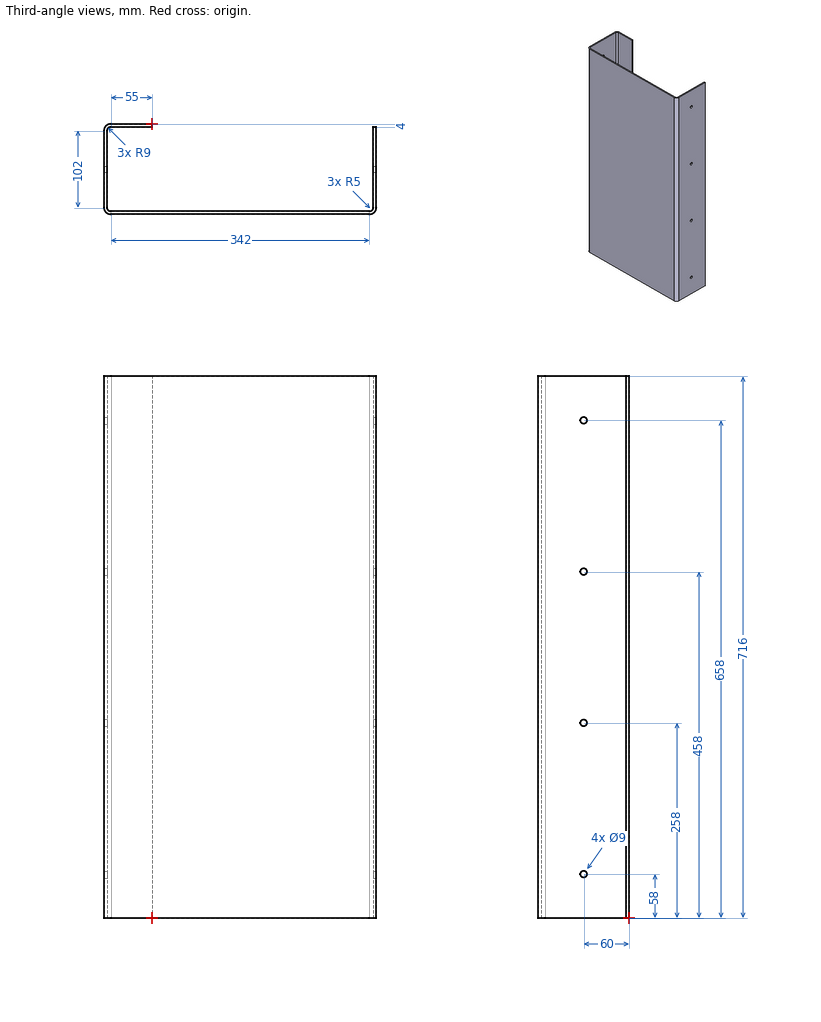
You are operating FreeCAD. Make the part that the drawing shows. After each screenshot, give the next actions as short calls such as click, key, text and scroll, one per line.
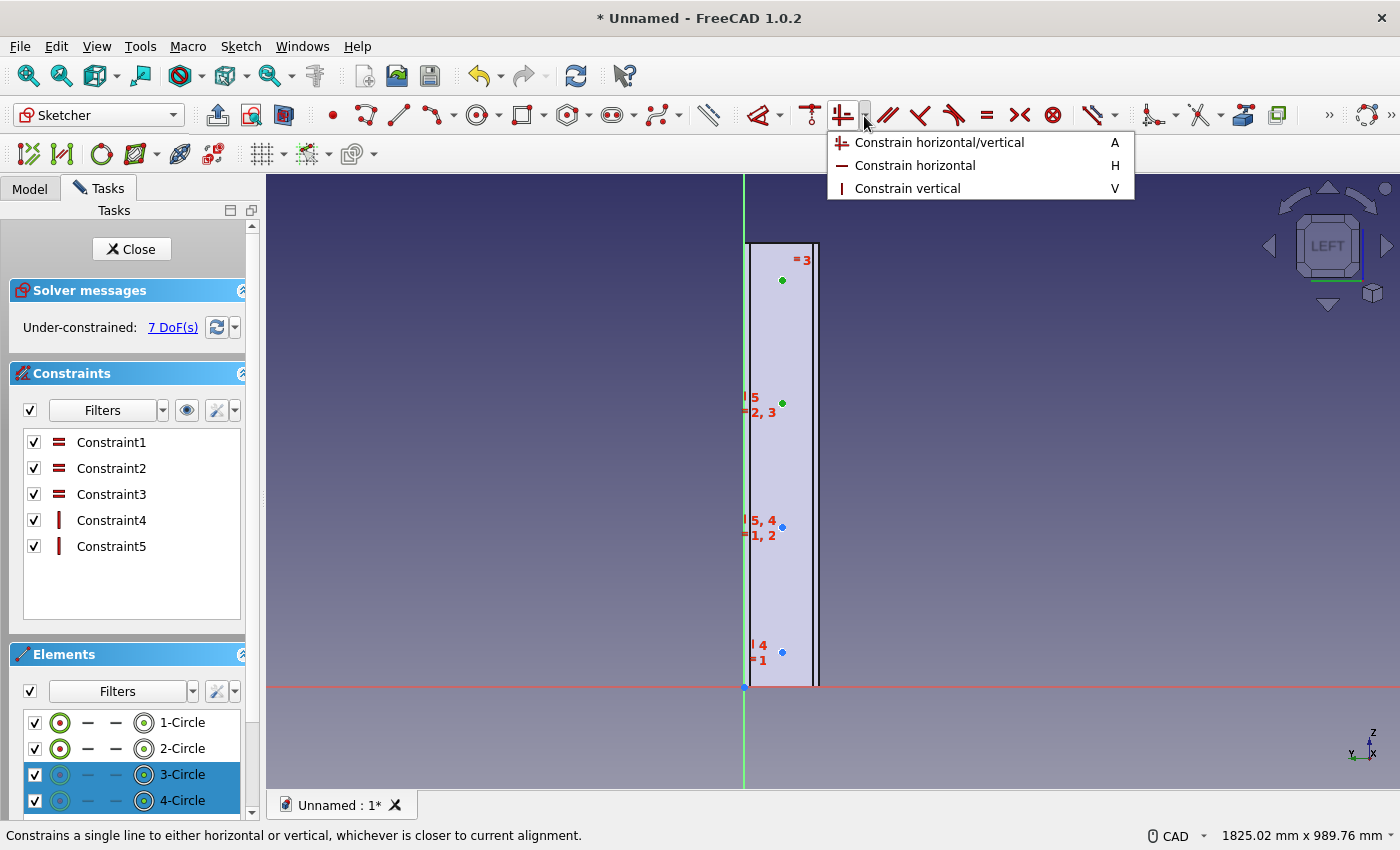
click(981, 188)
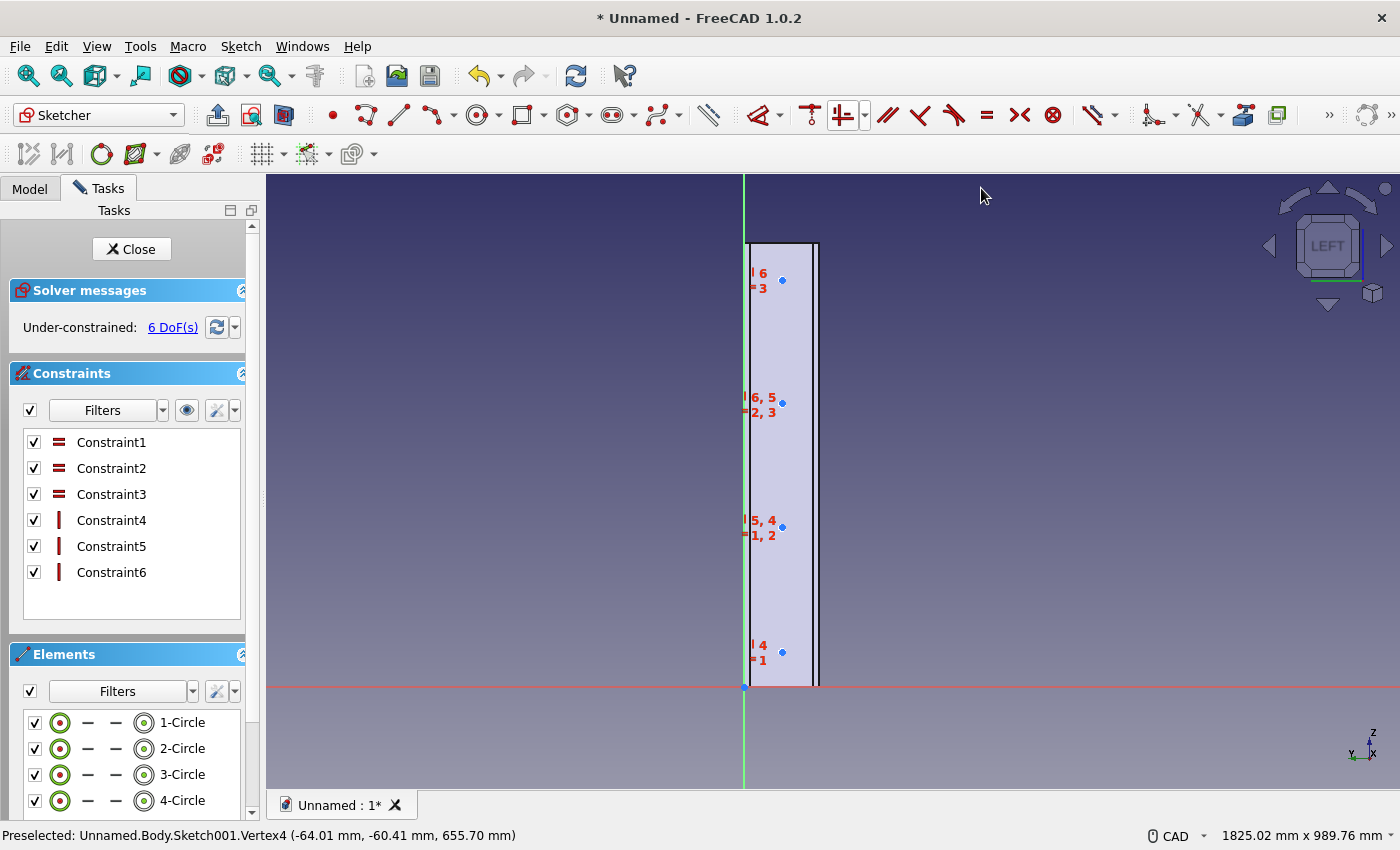
click(758, 116)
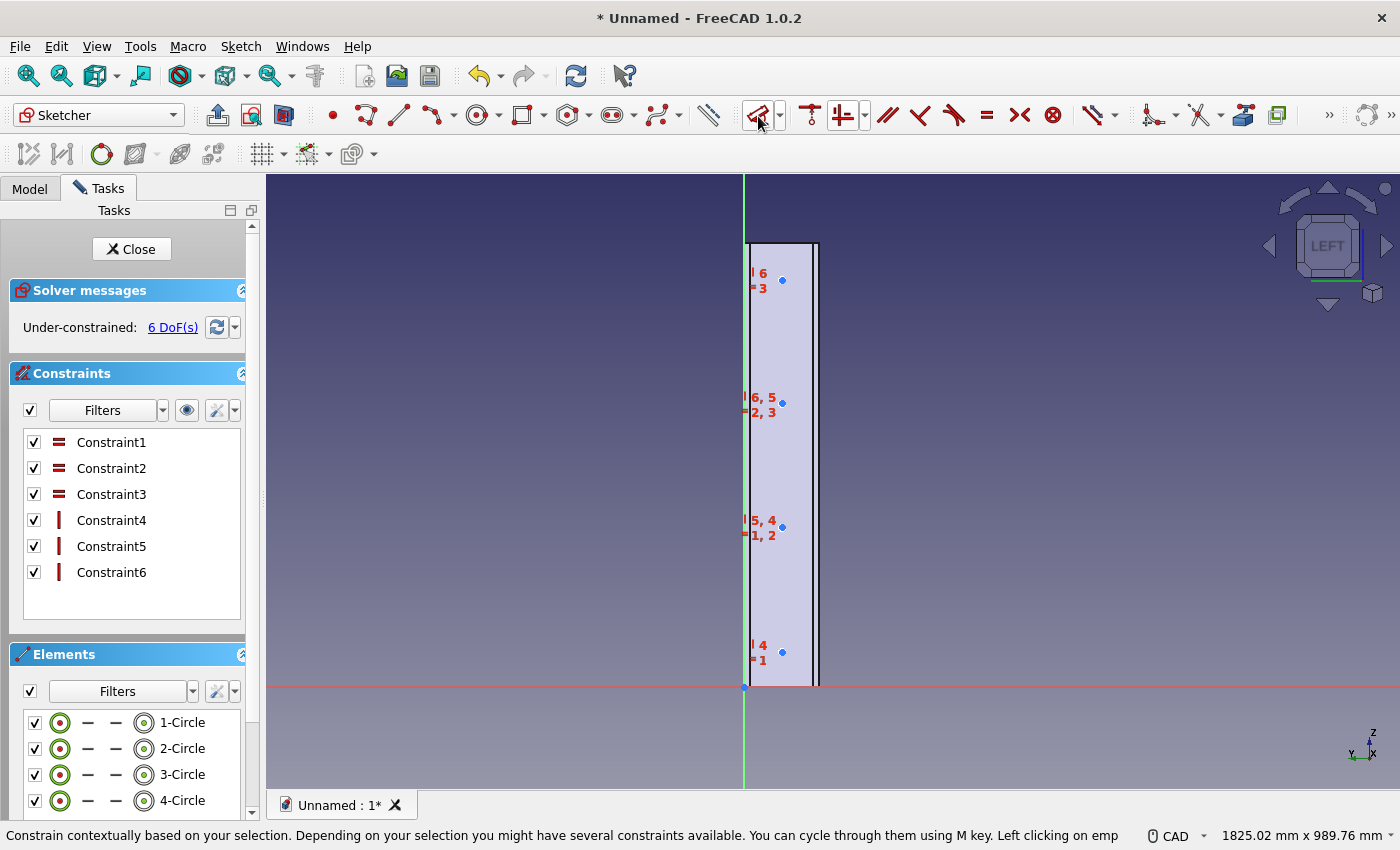
scroll(780, 650, up, 10)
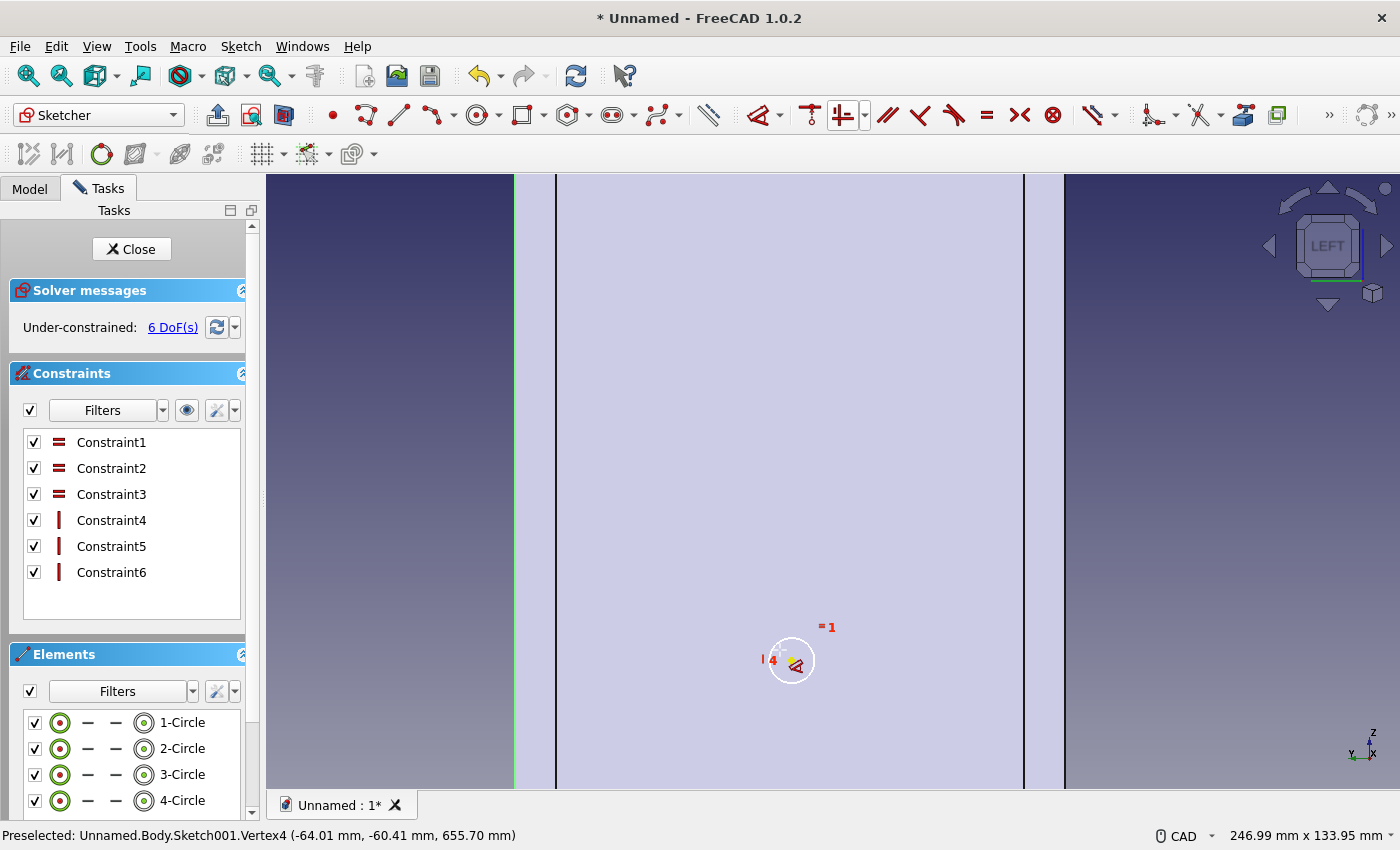
click(776, 645)
click(753, 623)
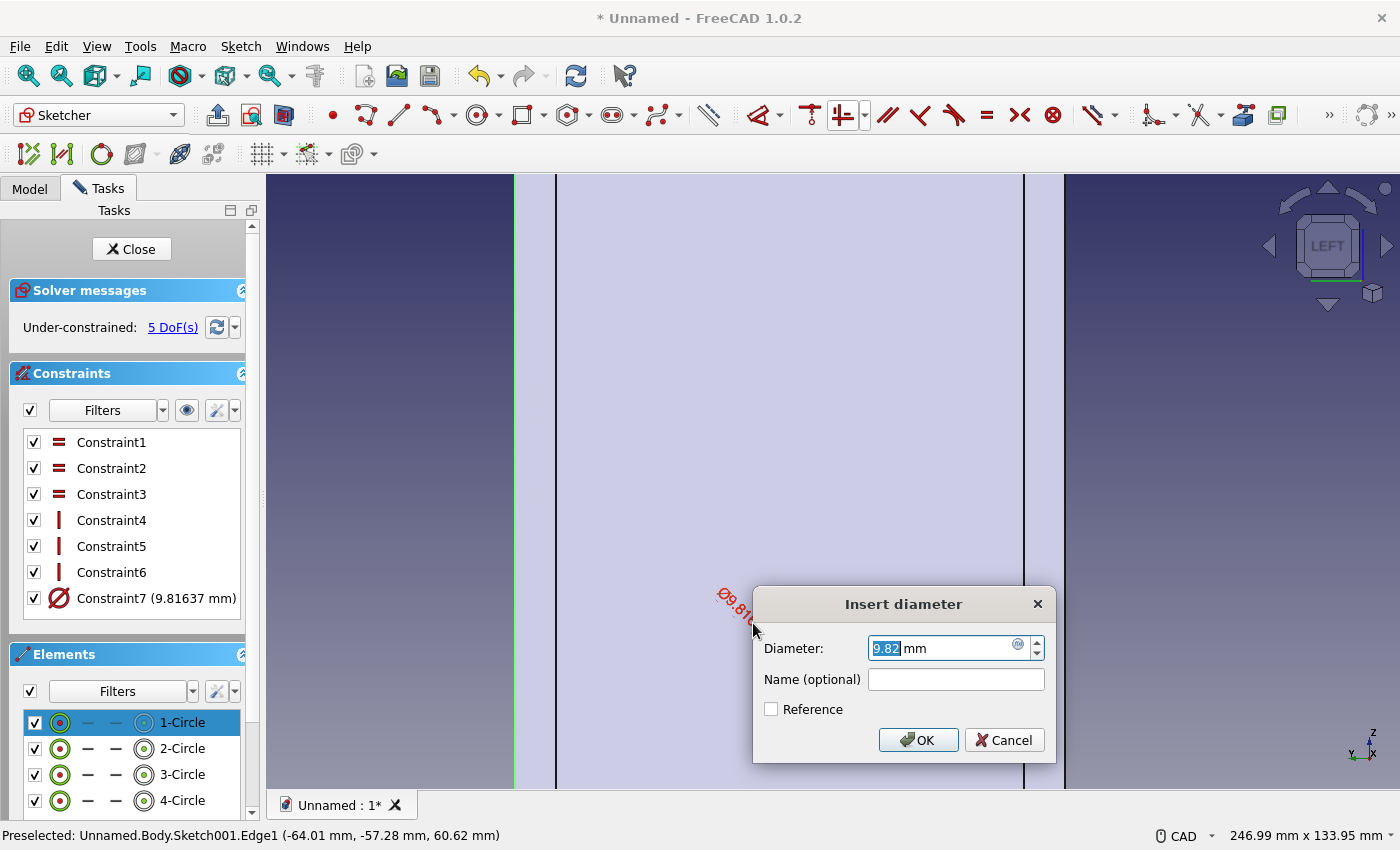
text(9)
key(Return)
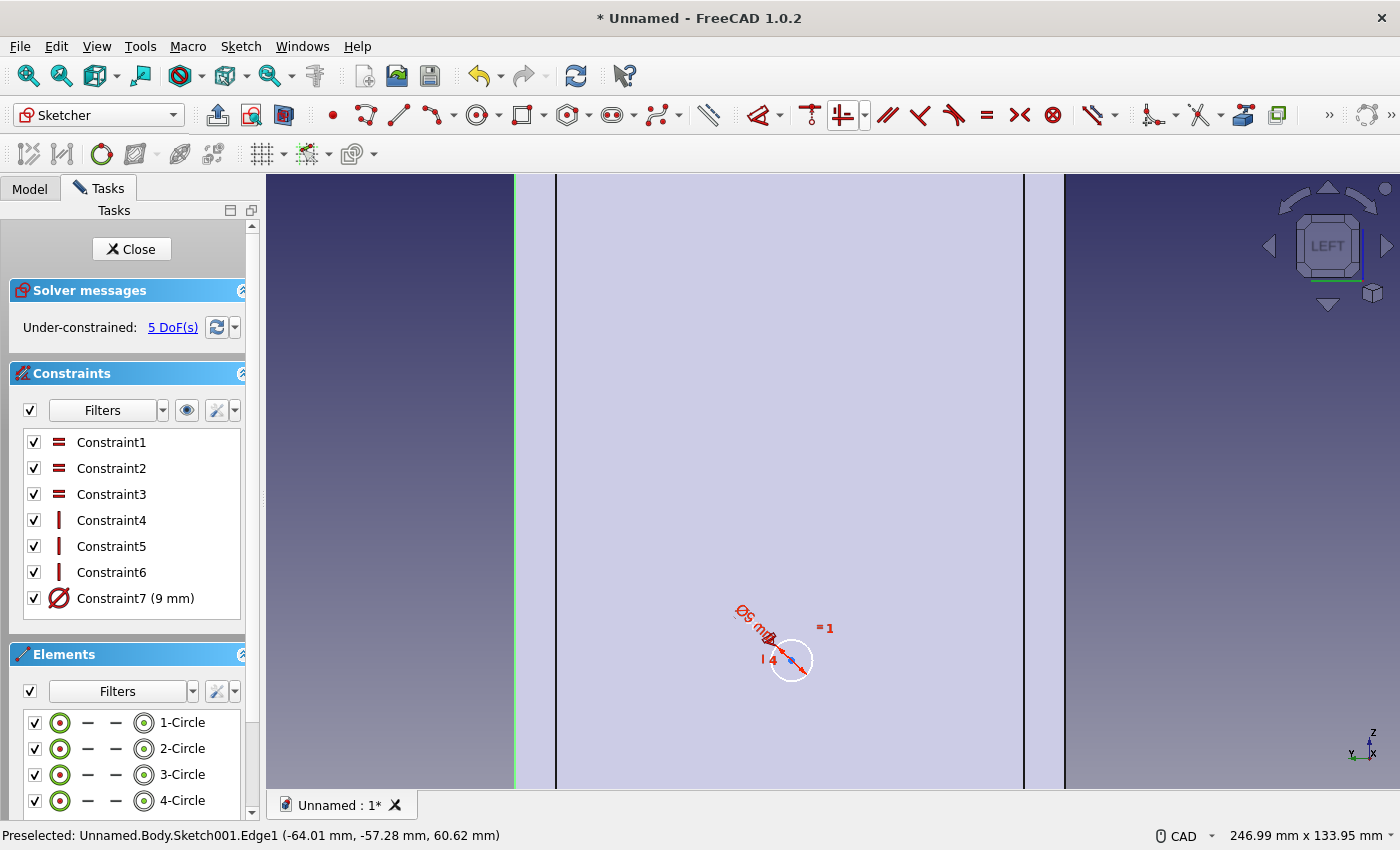
scroll(780, 651, down, 10)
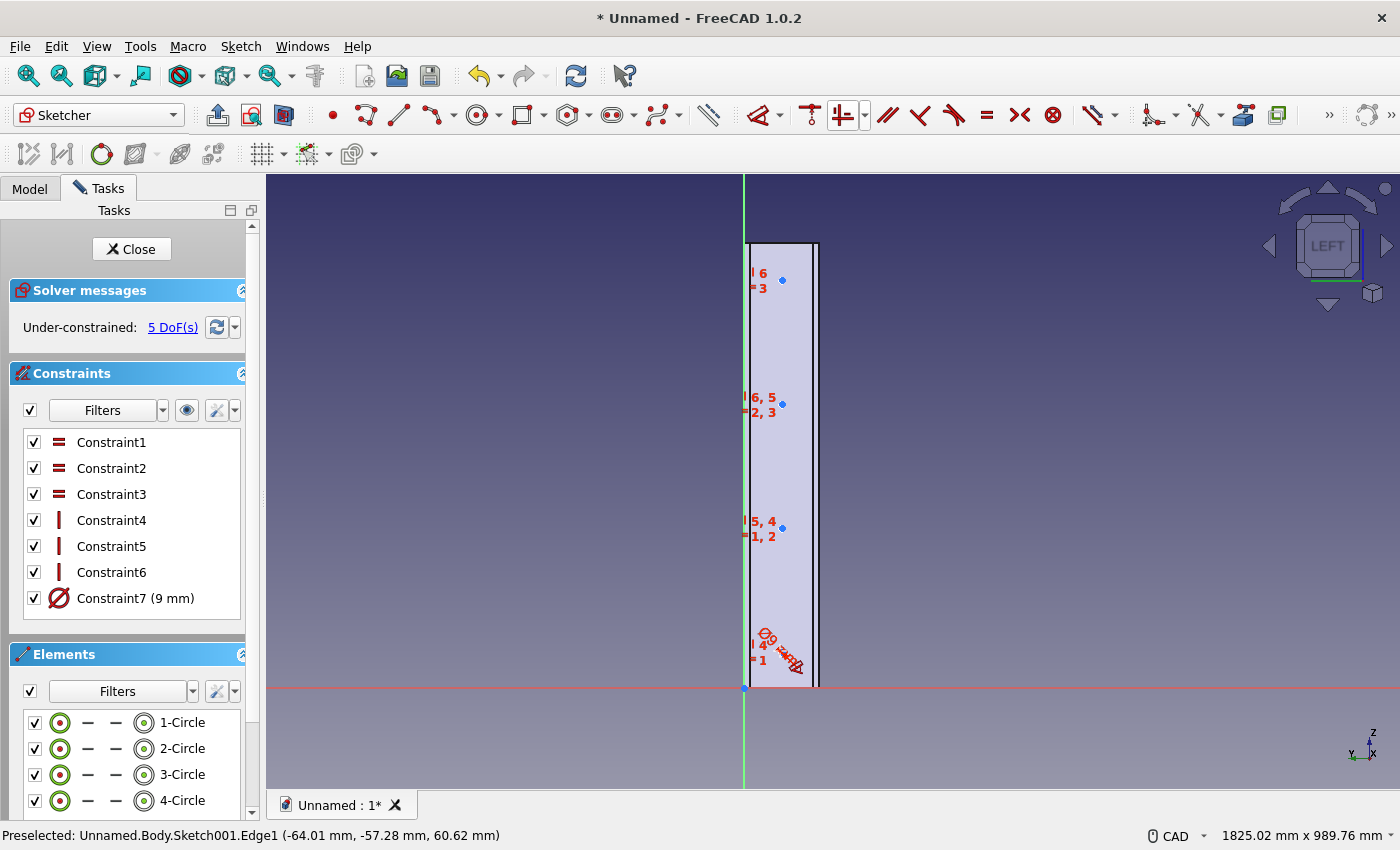
click(782, 653)
click(763, 722)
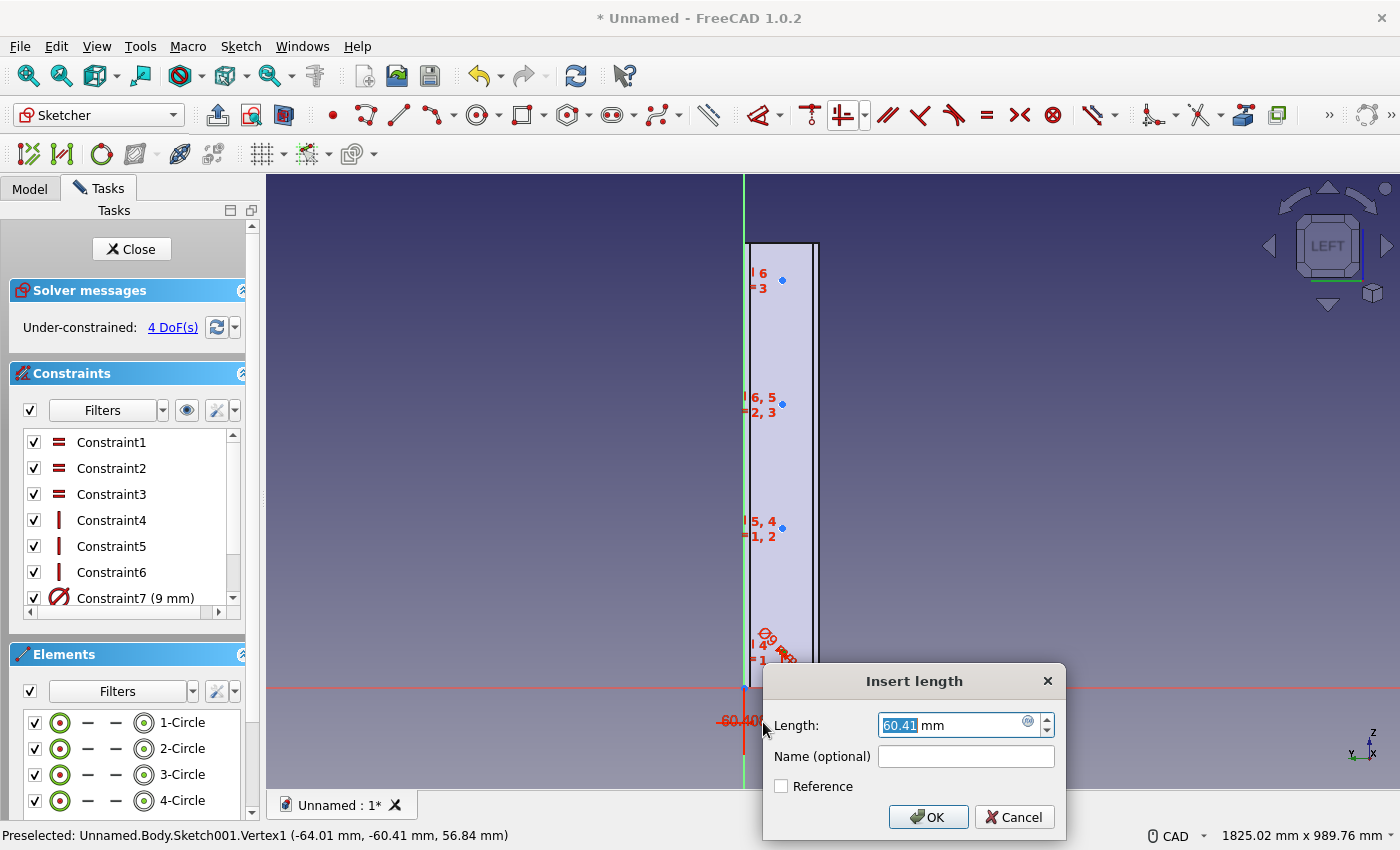
text(60)
key(Return)